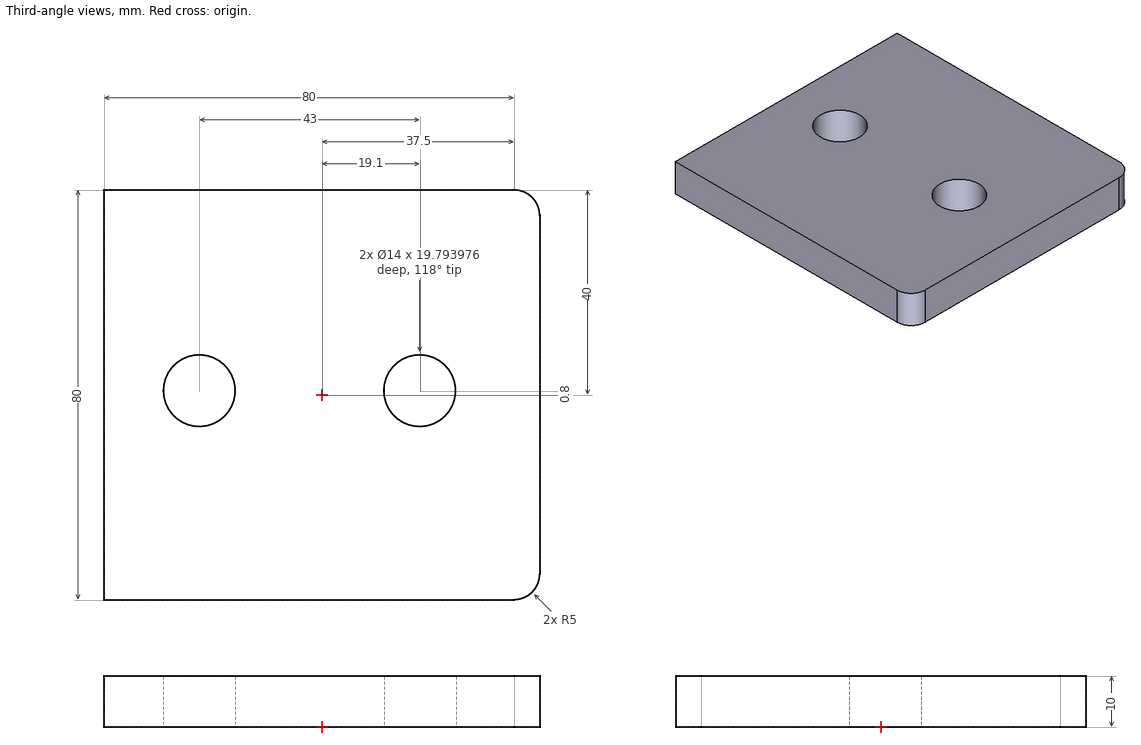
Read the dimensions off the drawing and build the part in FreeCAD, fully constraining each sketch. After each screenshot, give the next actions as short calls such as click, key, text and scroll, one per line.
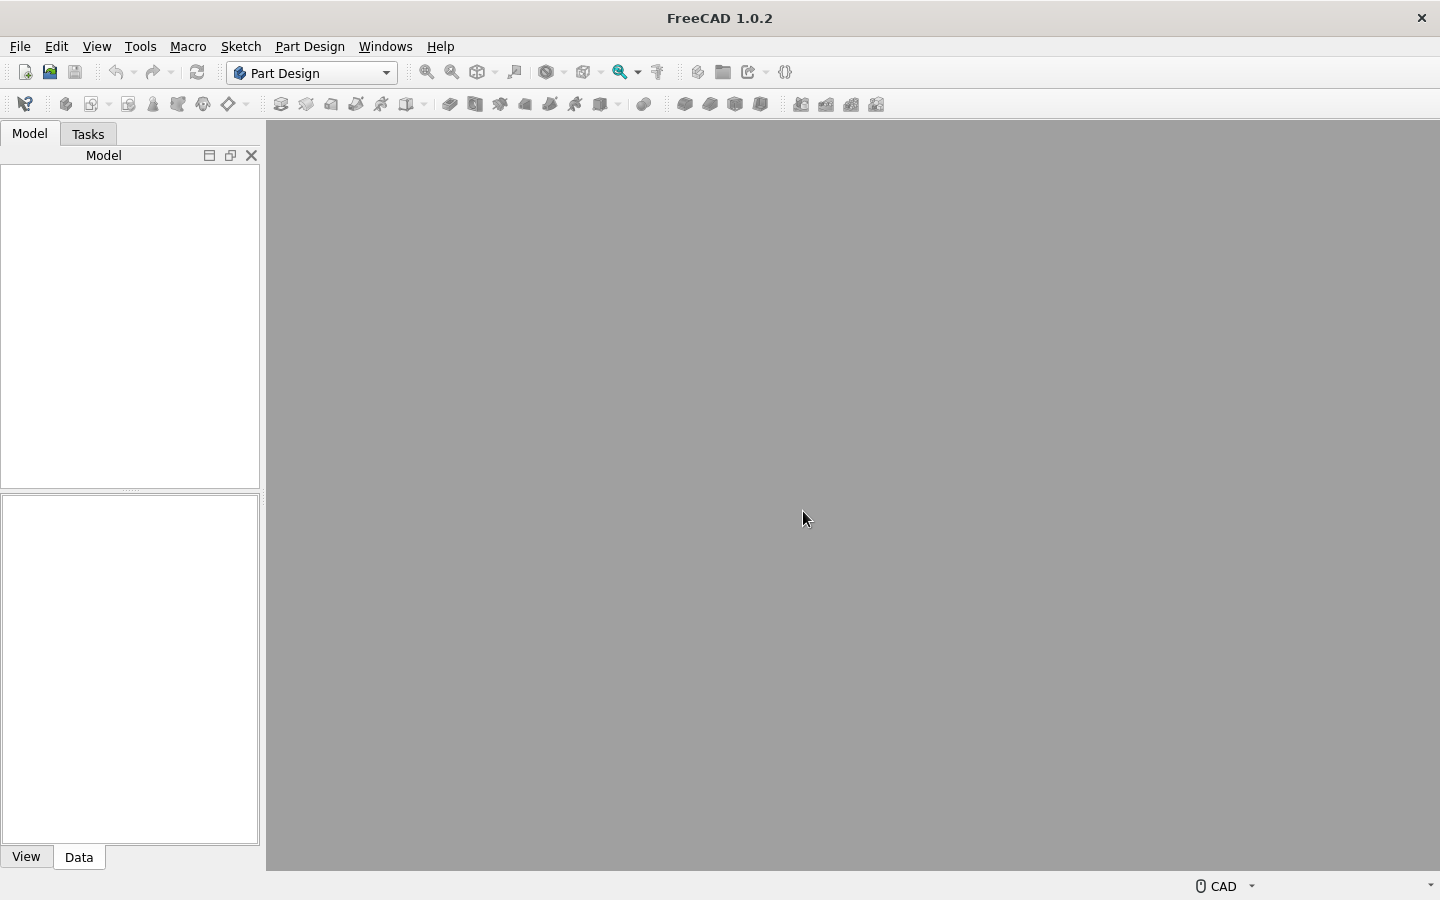
click(25, 72)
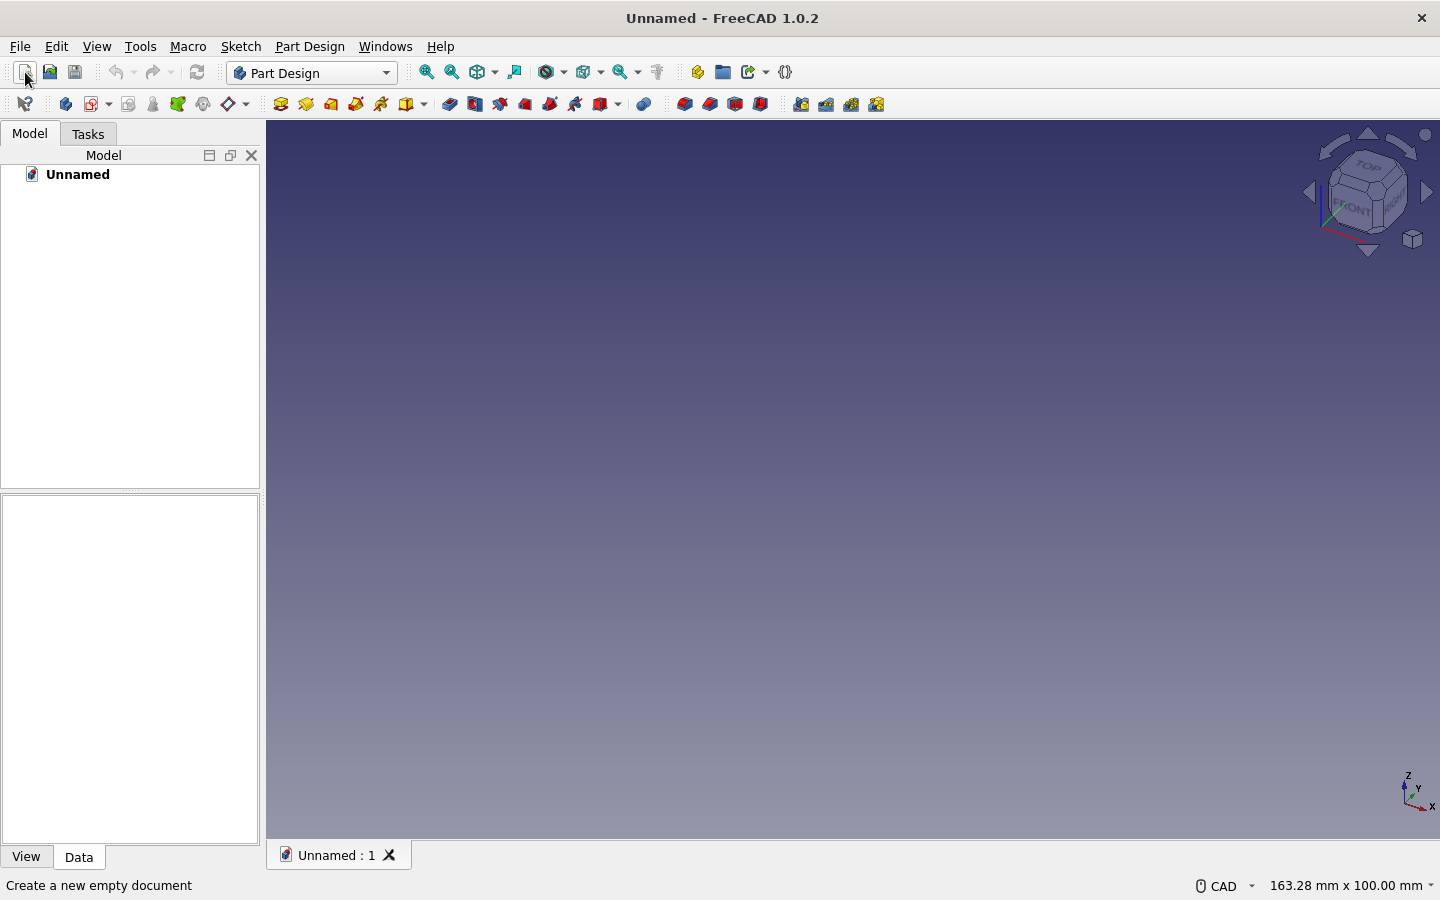
click(90, 104)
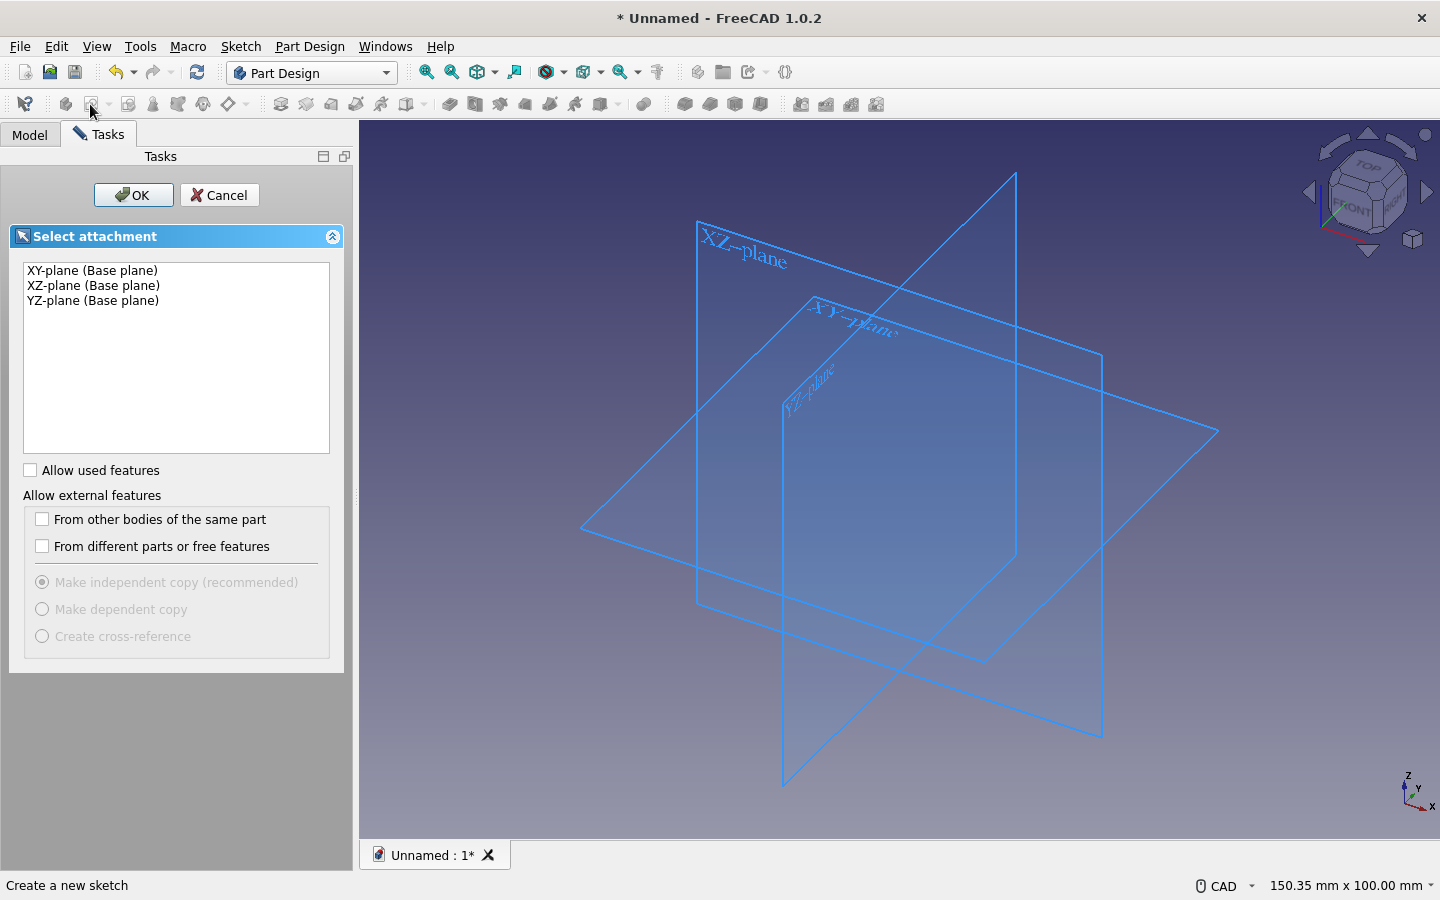
click(84, 270)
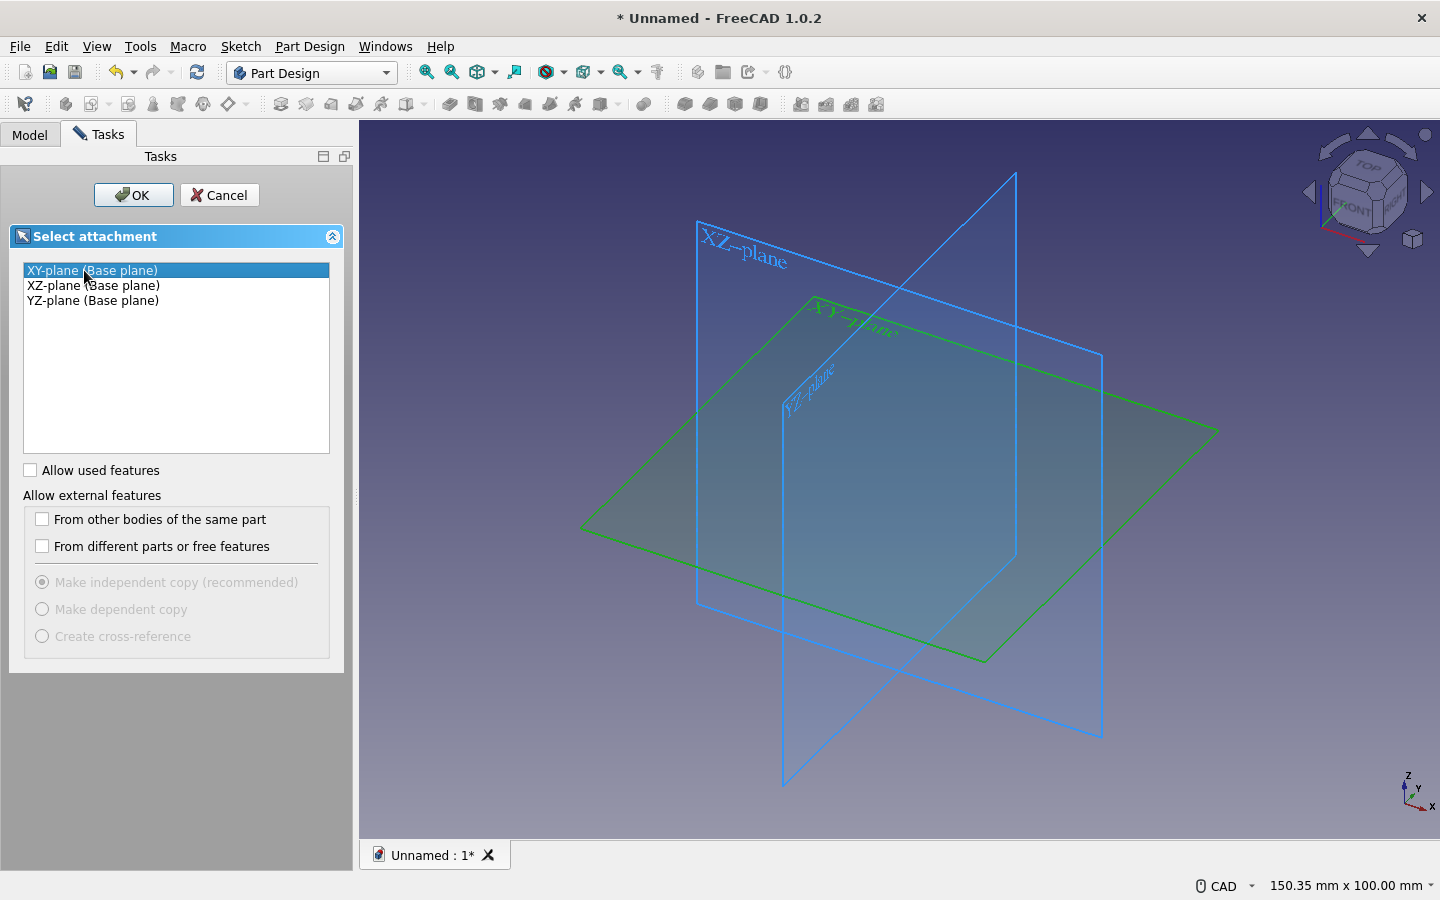
click(134, 195)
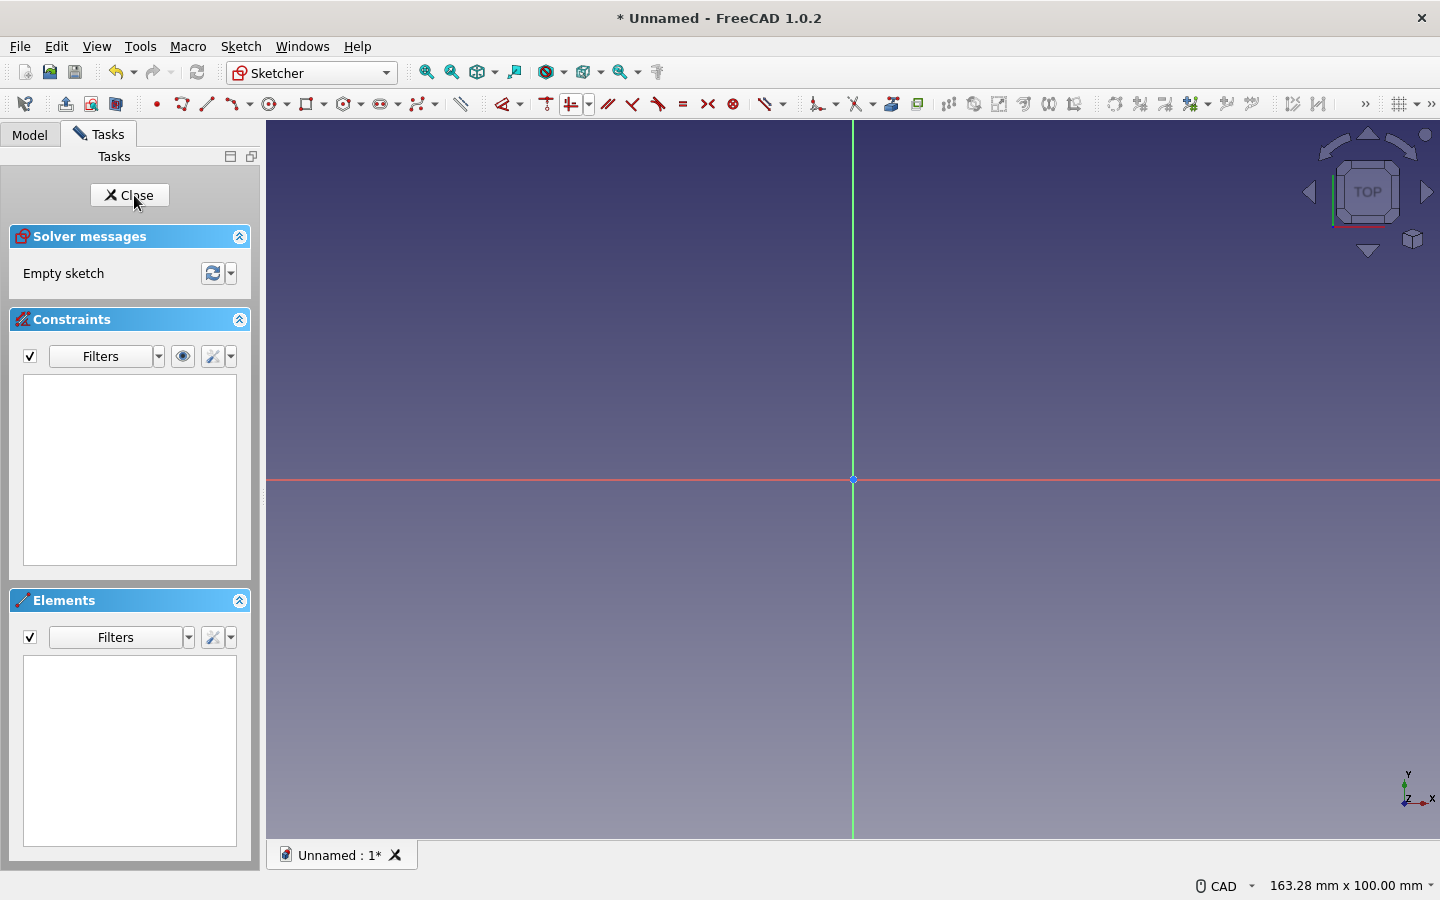
click(182, 104)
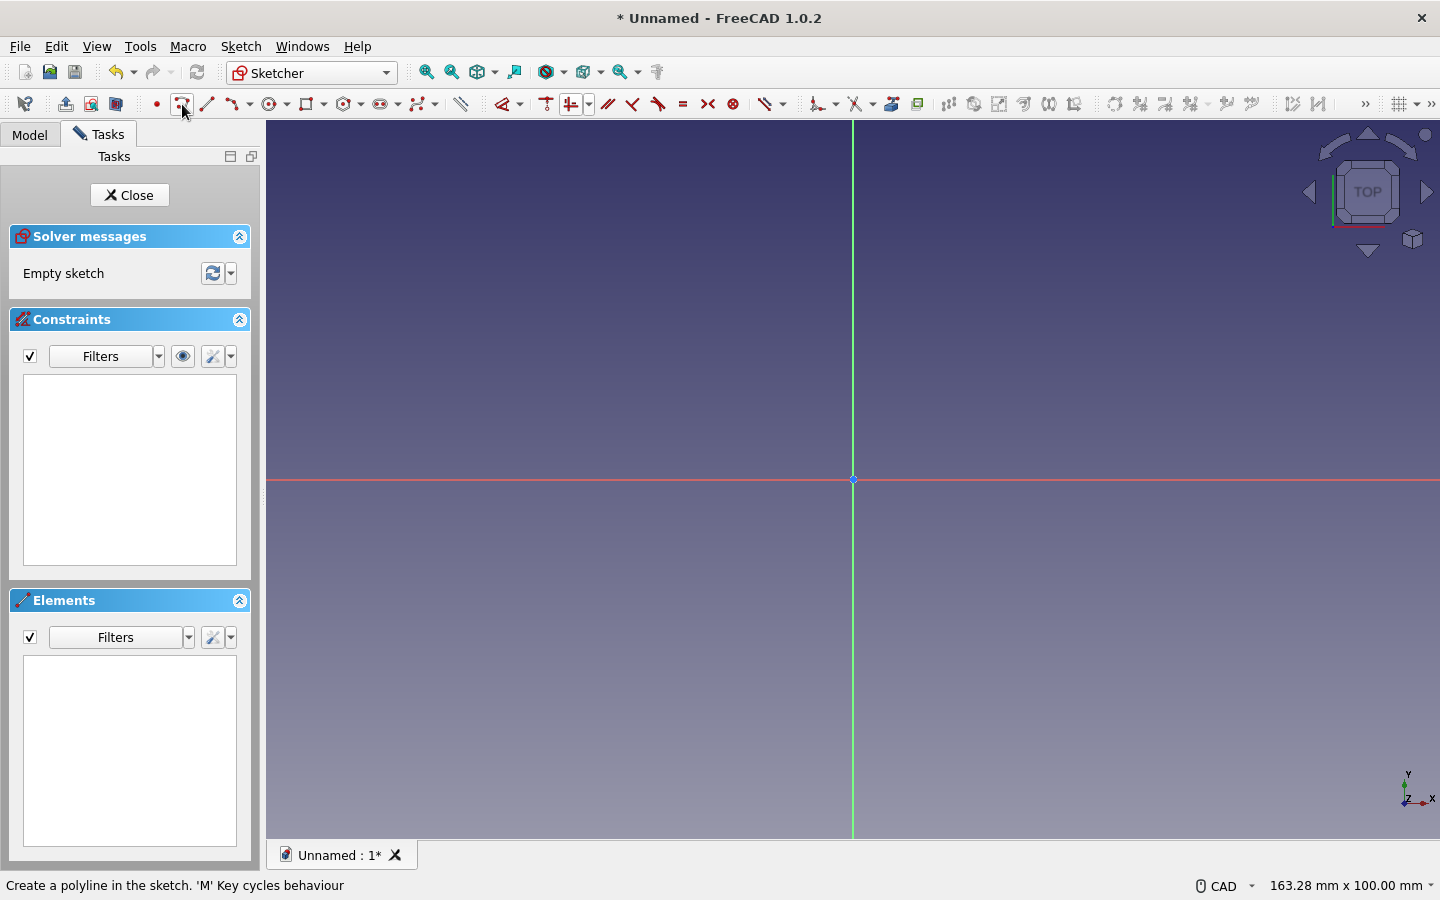
click(1123, 192)
click(547, 192)
click(547, 767)
click(1123, 767)
right_click(1123, 767)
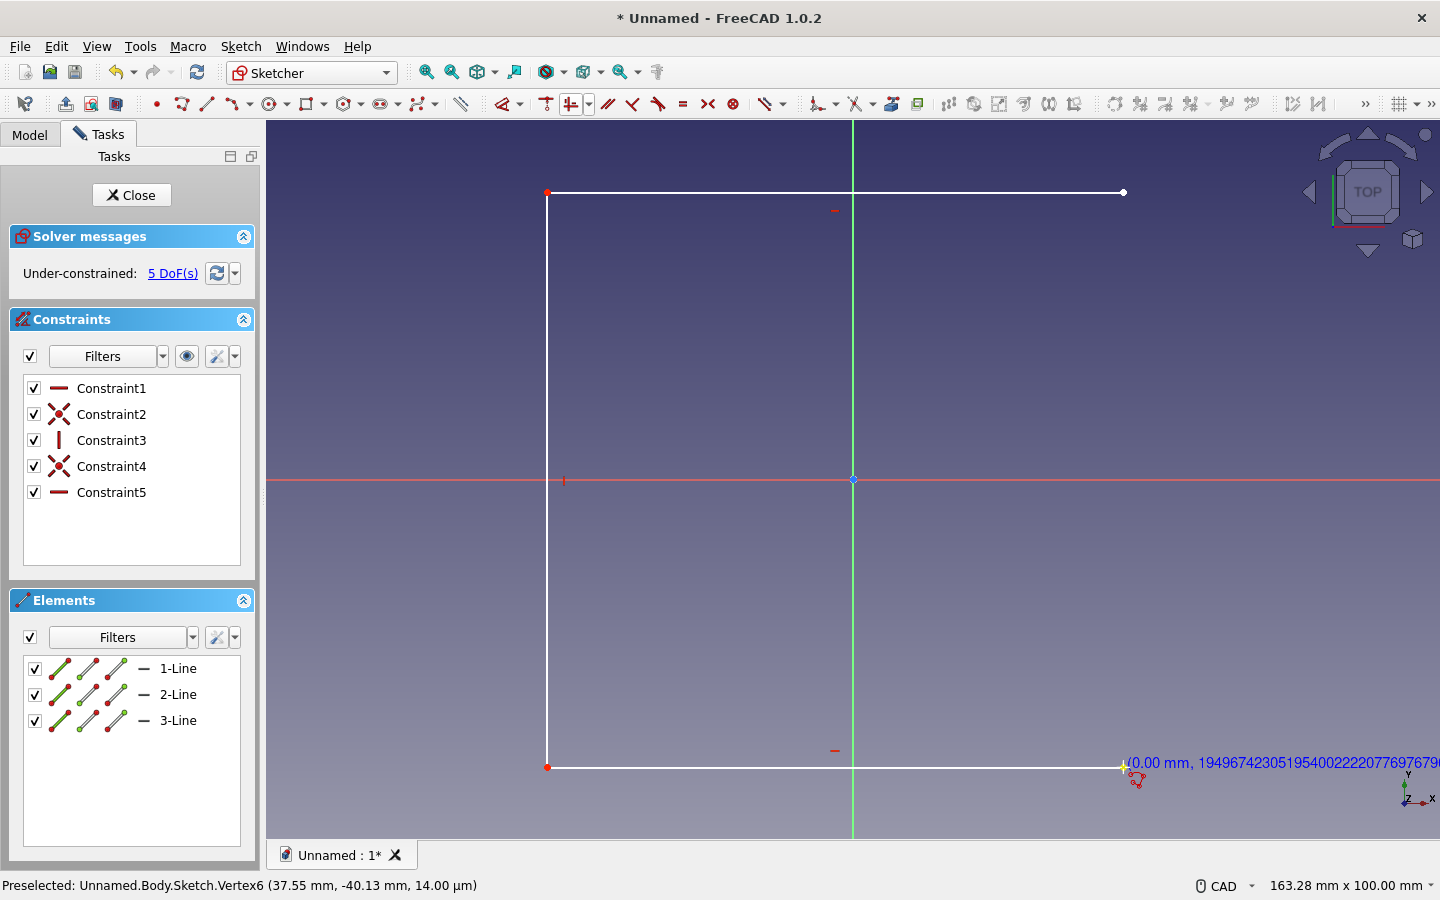
click(207, 104)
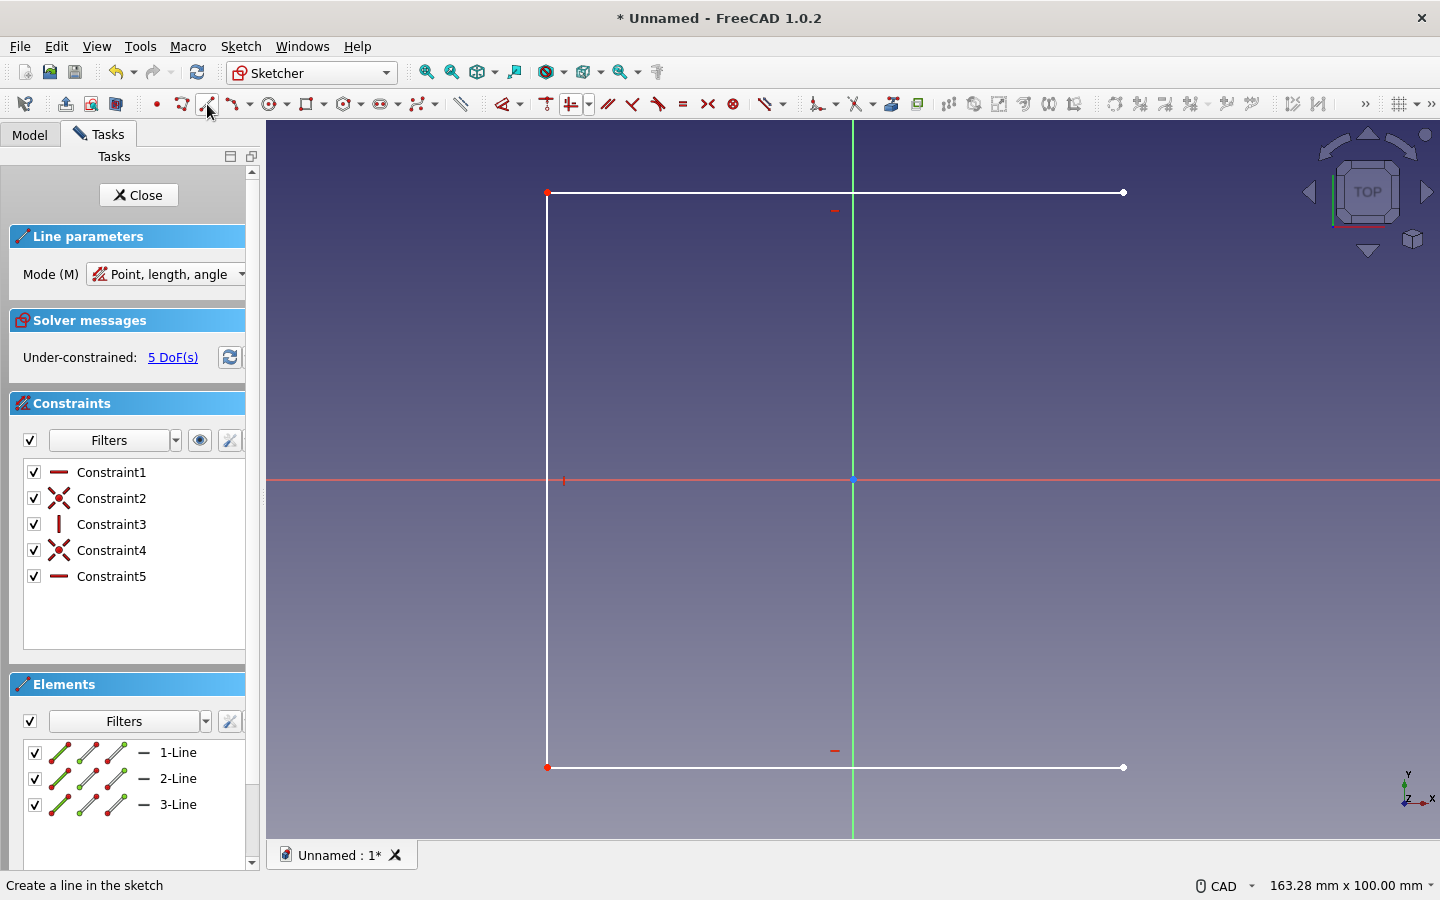
click(1159, 731)
click(1159, 228)